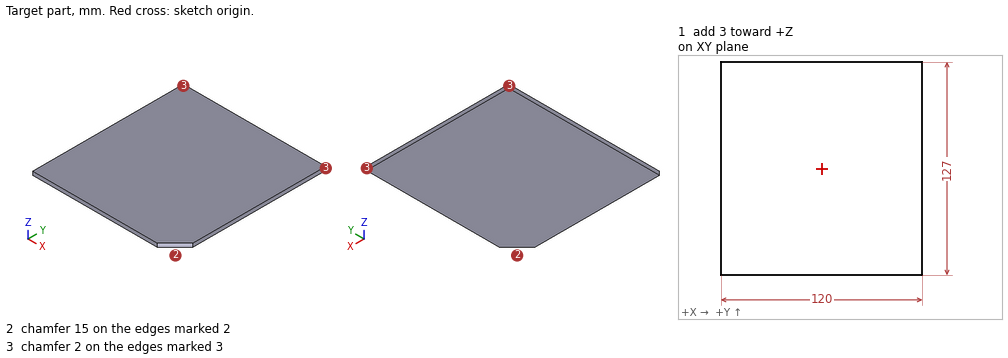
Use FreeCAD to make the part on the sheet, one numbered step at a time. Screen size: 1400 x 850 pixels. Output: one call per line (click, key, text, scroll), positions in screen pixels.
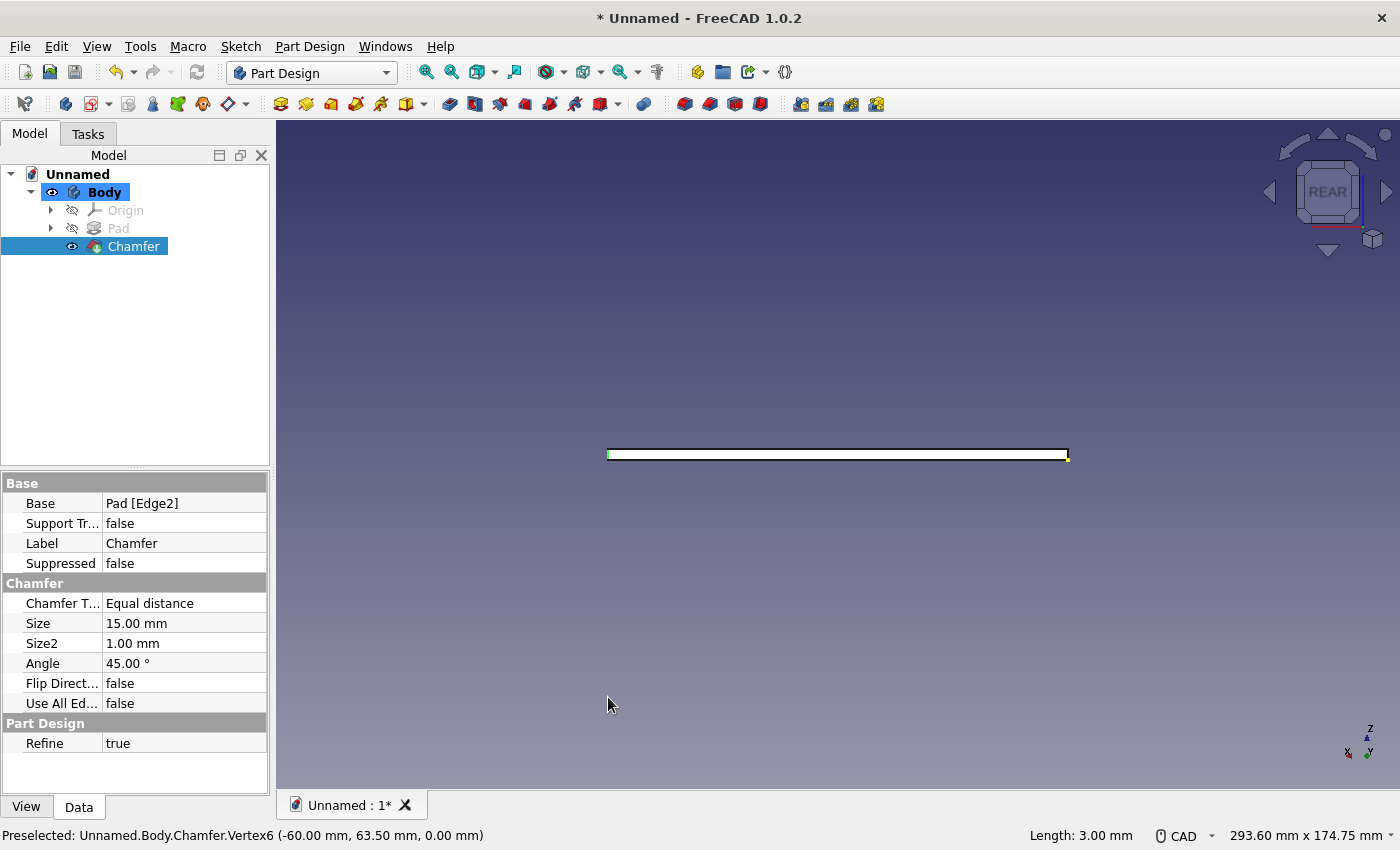
scroll(1068, 454, up, 7)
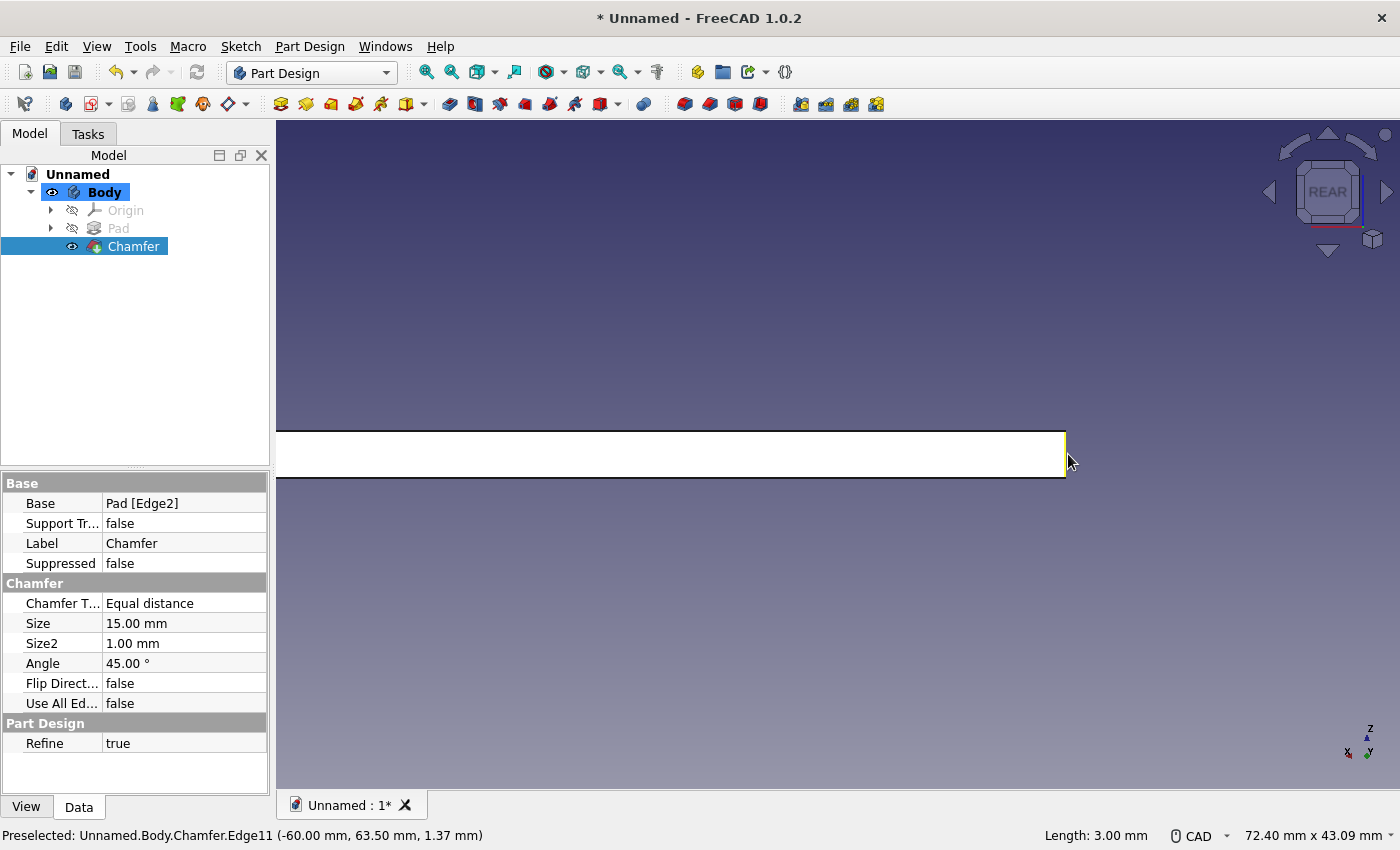
click(1065, 454, ctrl)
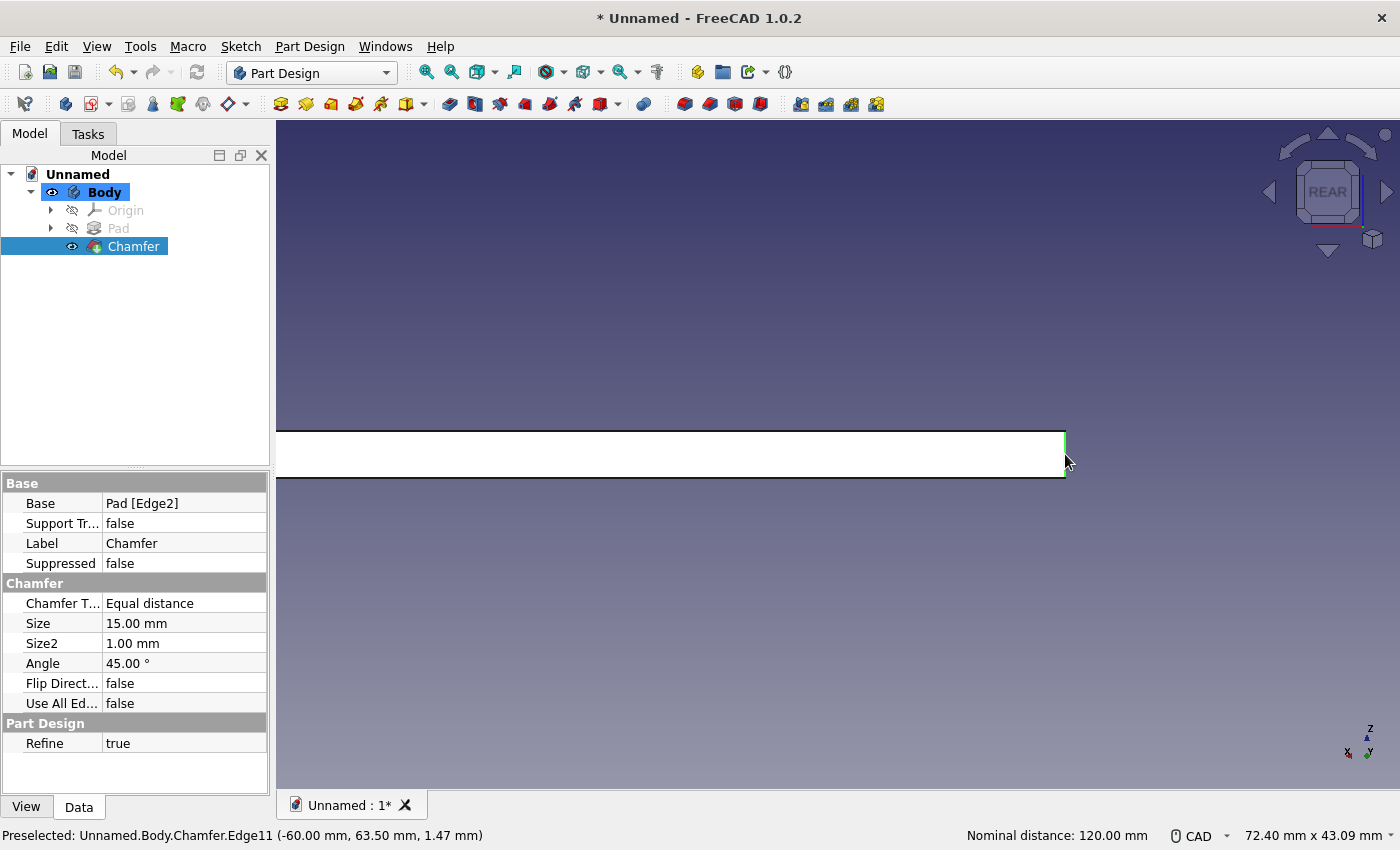
click(710, 104)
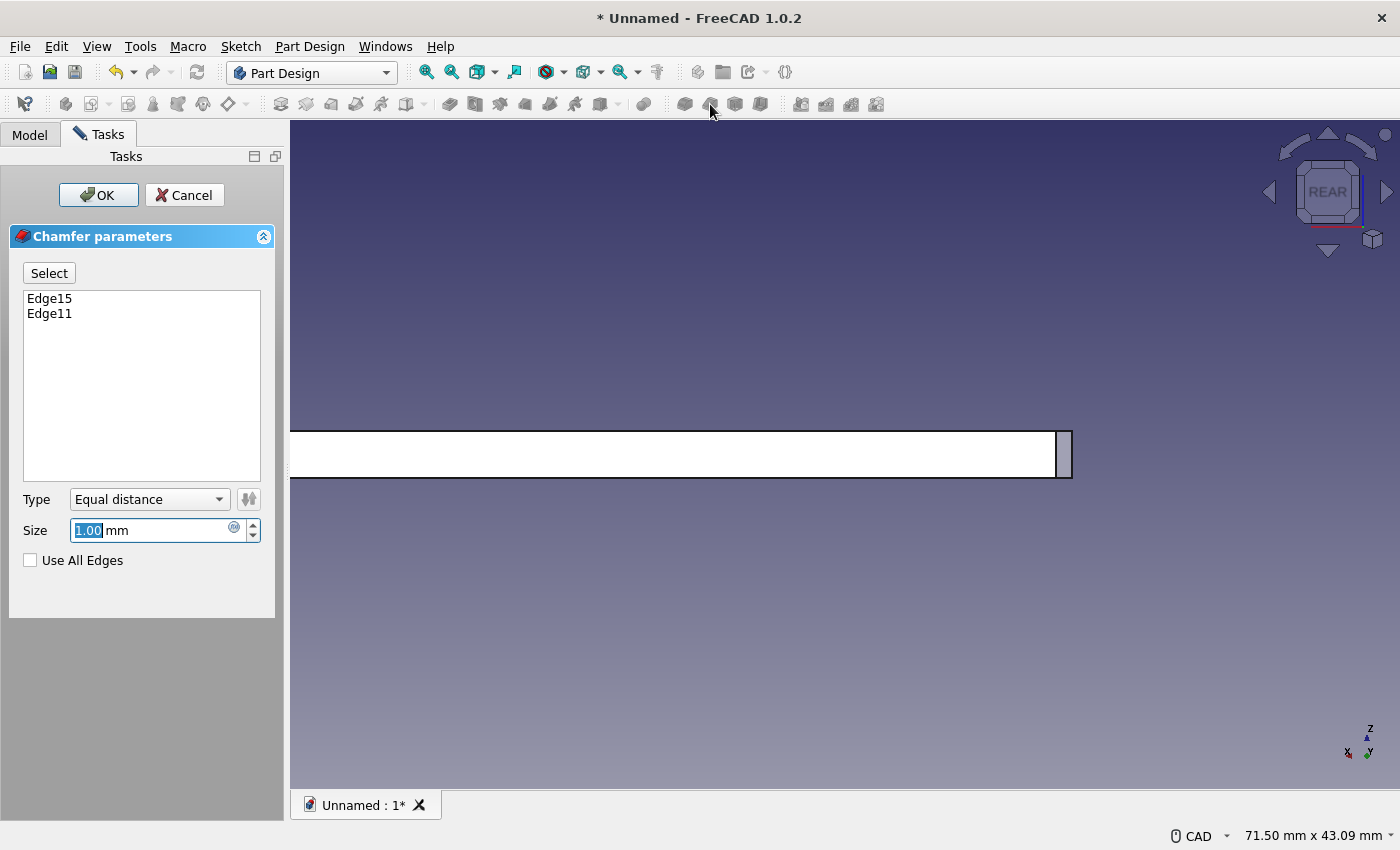
text(2)
key(Tab)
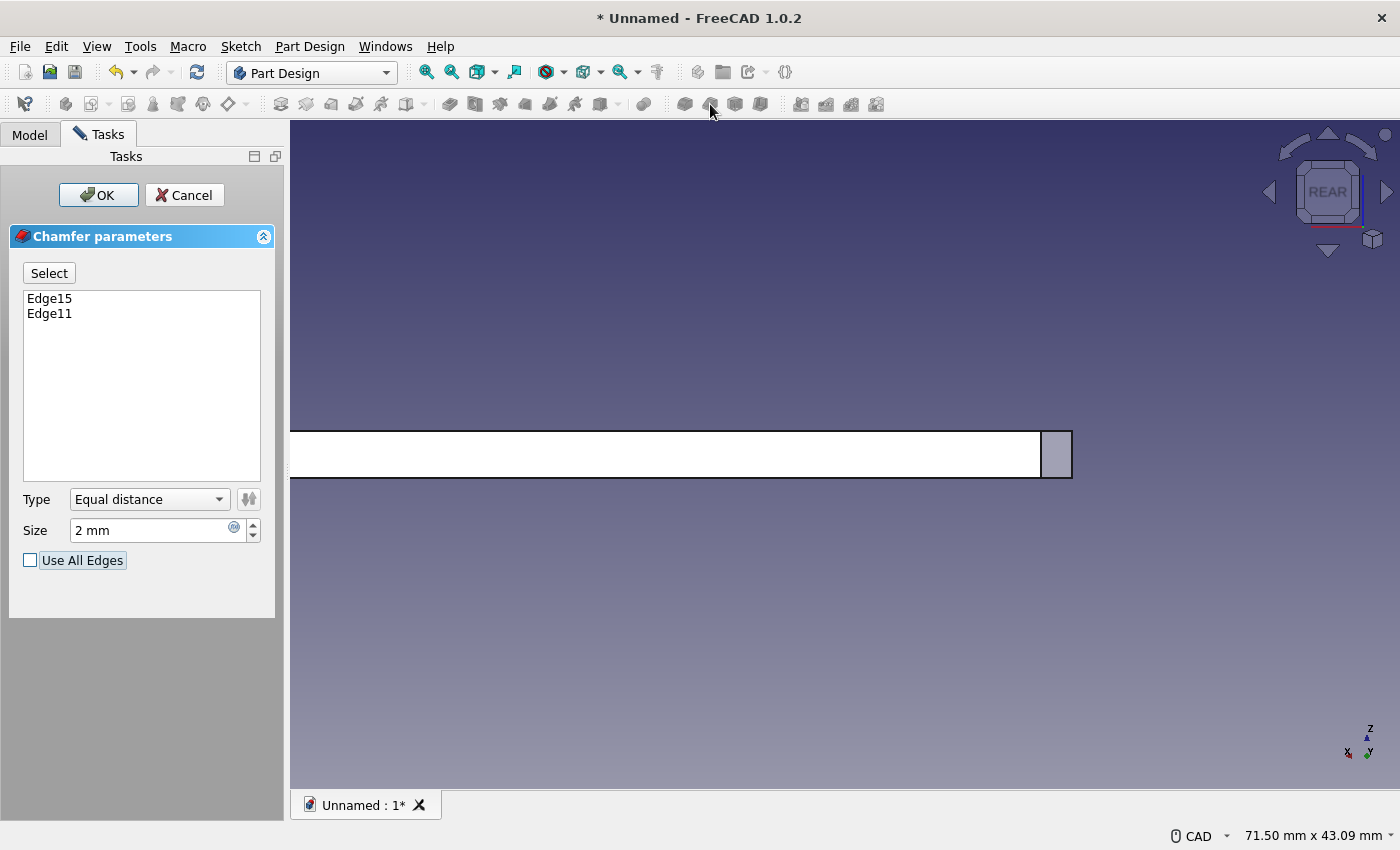
click(99, 195)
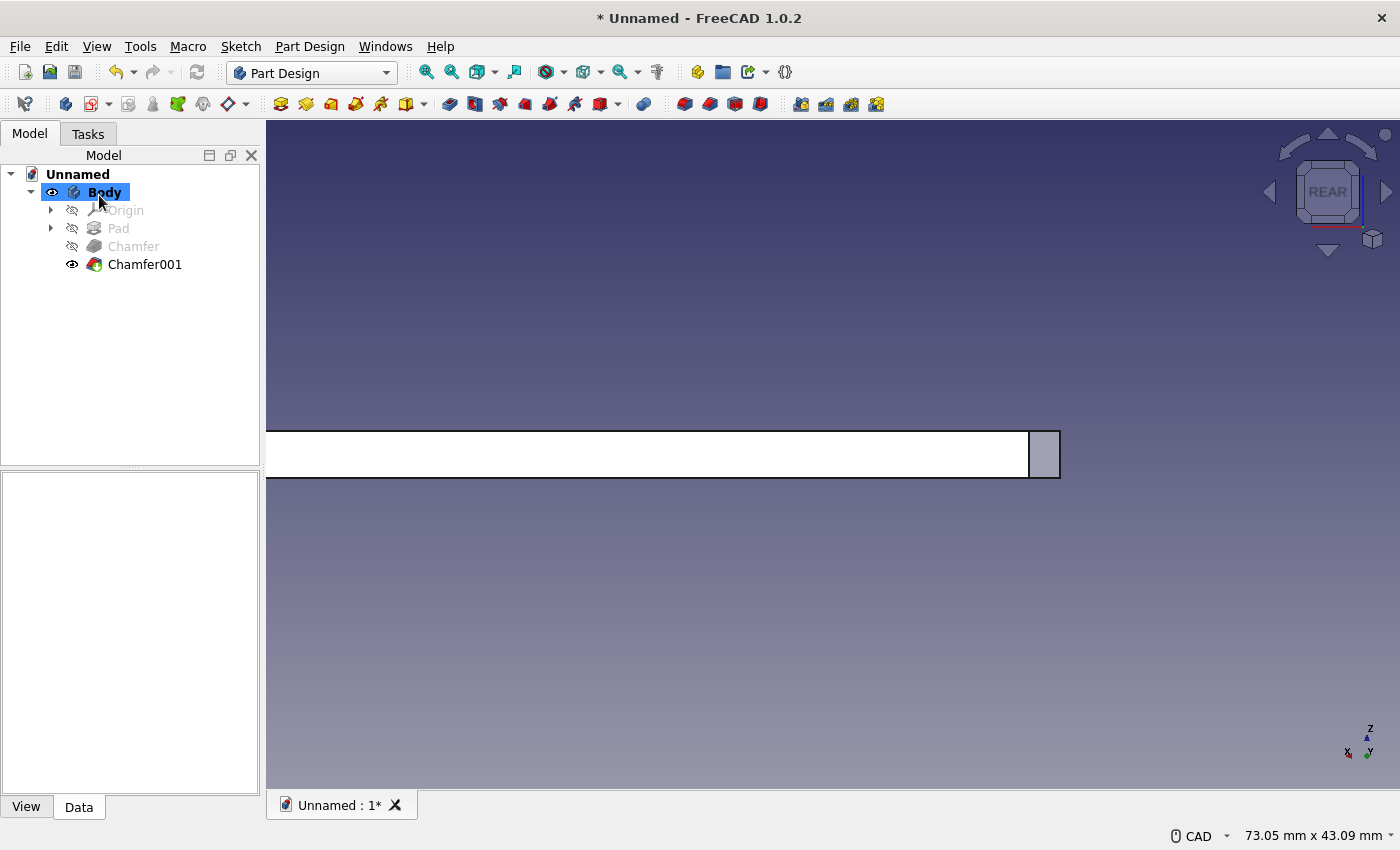
key(0)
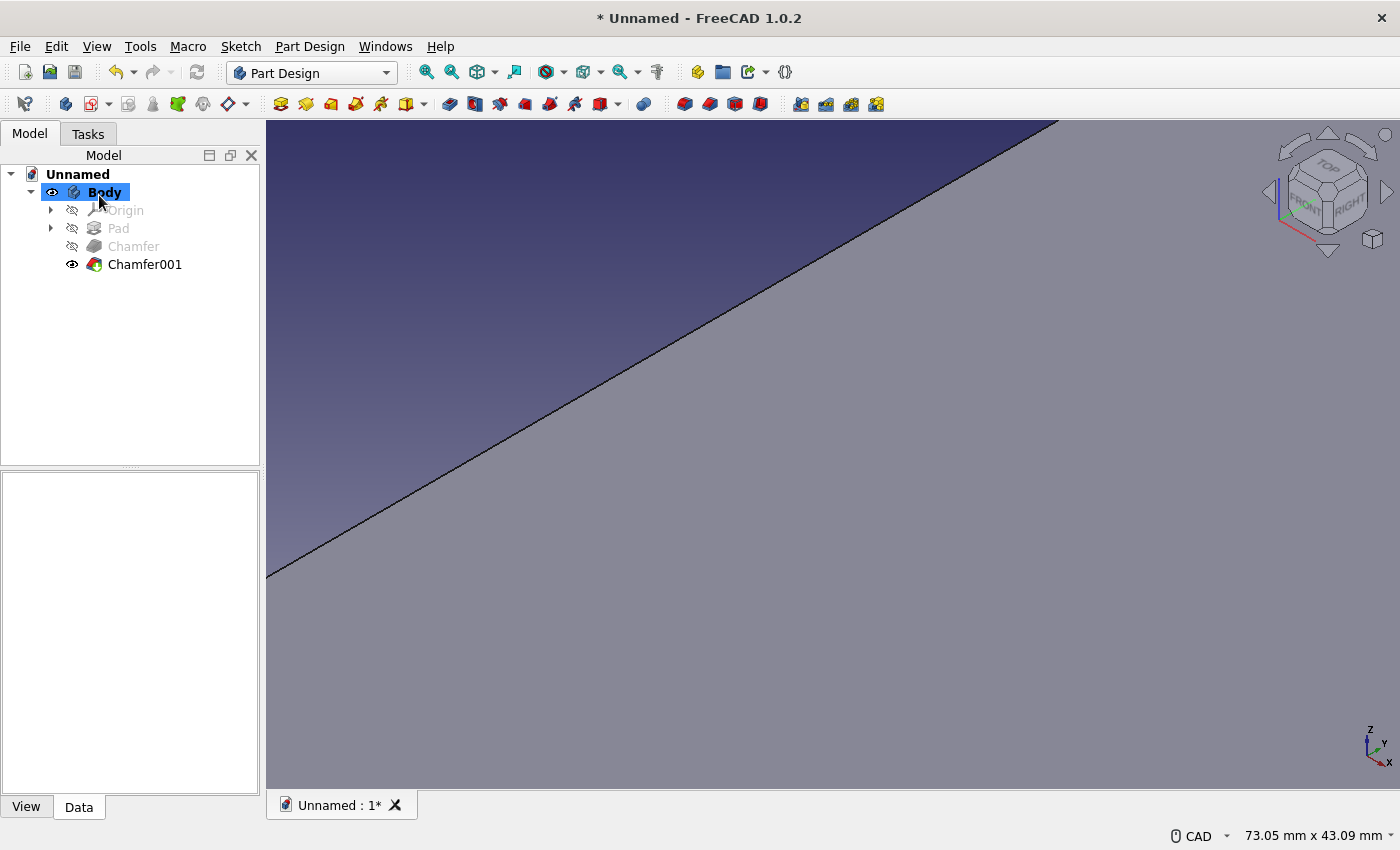
key(v)
key(f)